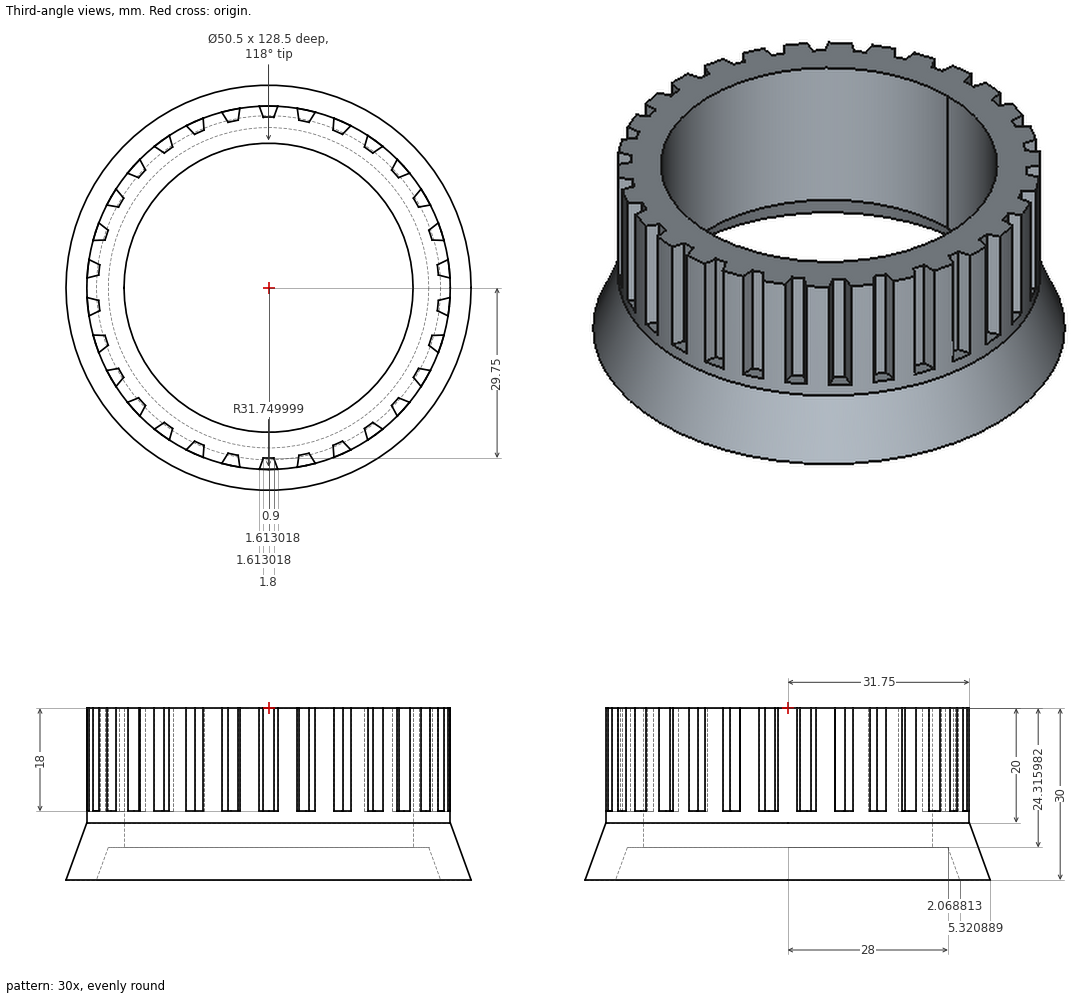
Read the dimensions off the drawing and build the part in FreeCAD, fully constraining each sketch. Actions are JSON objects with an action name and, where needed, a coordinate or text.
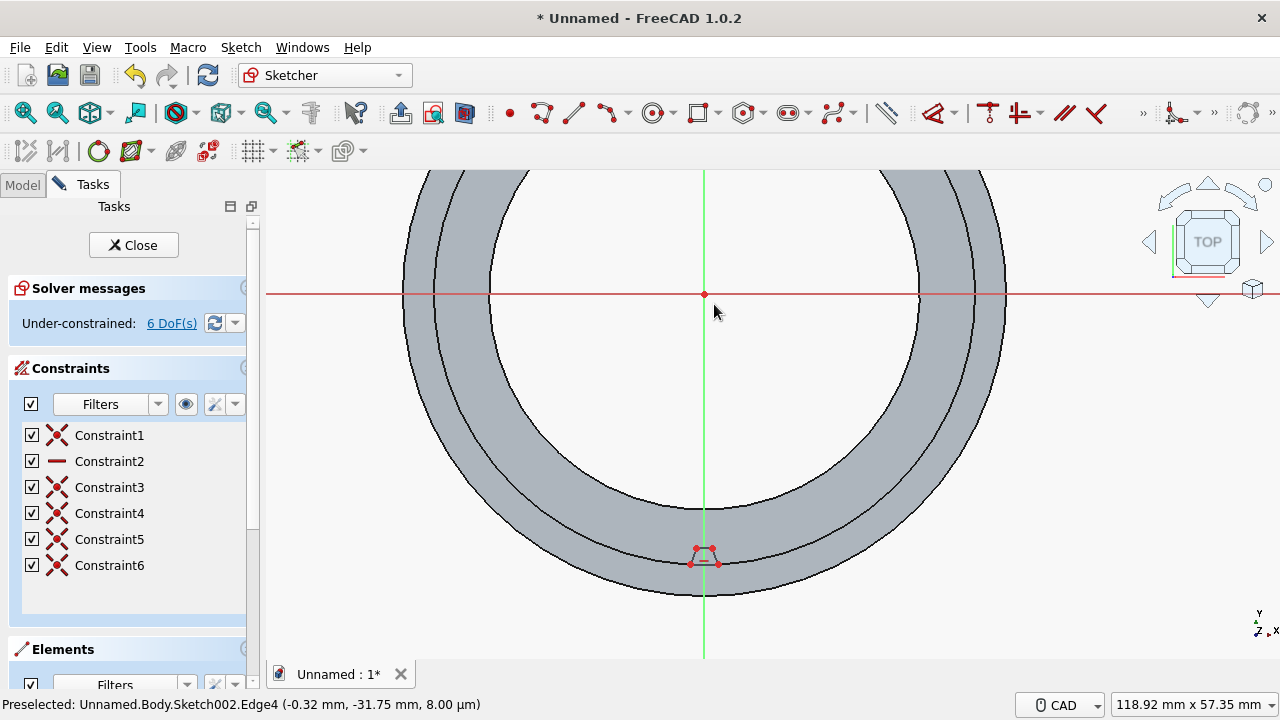
{"action": "left_click", "coordinate": [934, 114]}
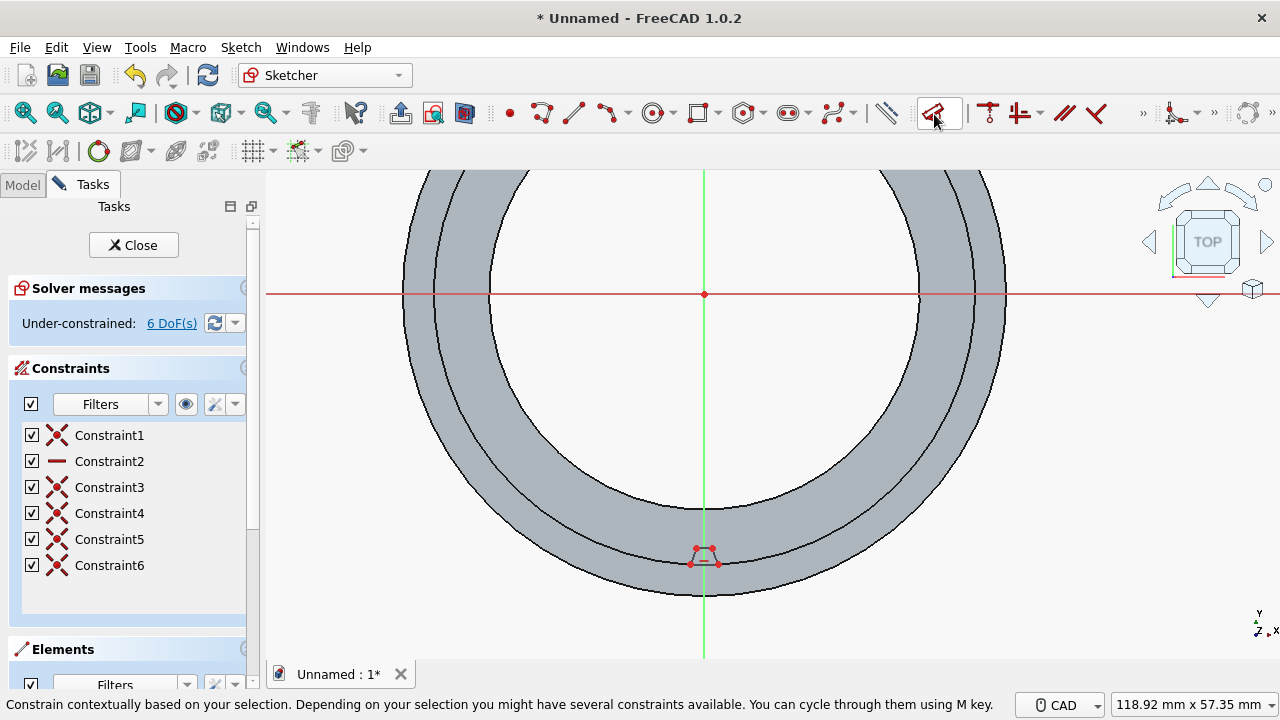
{"action": "left_click", "coordinate": [704, 565]}
{"action": "left_click", "coordinate": [559, 560]}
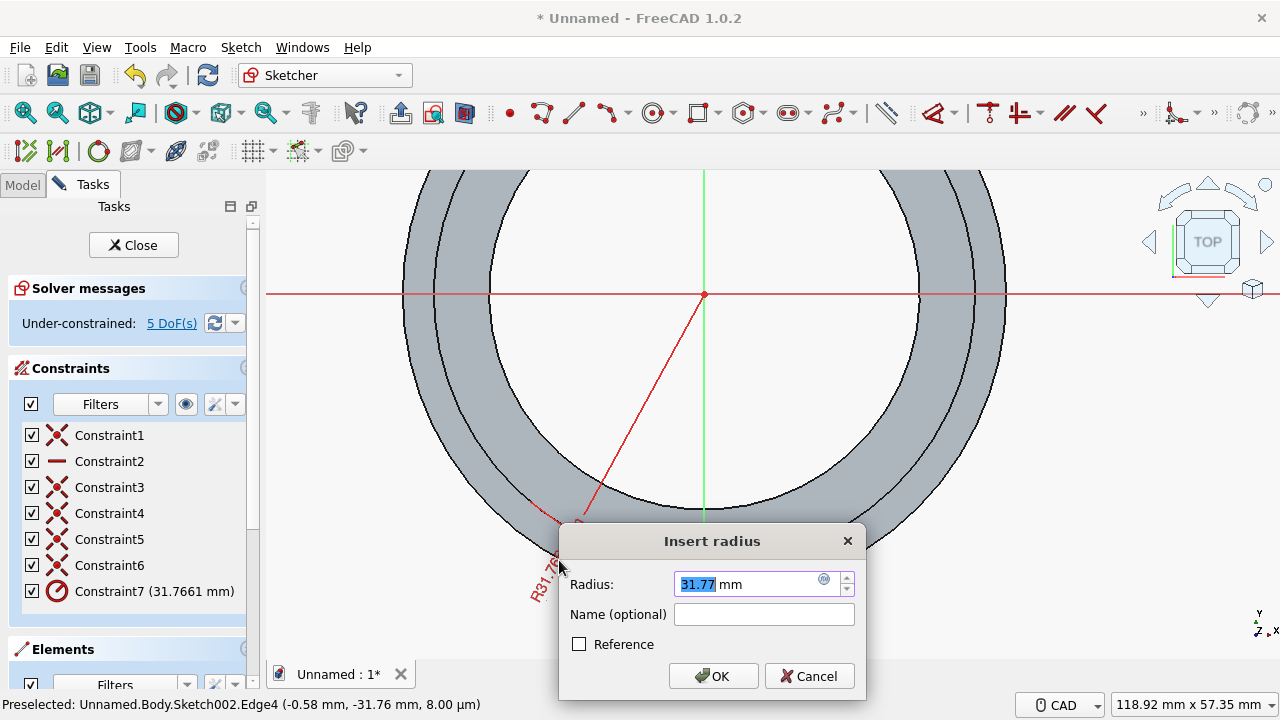
{"action": "type", "text": "31.749999"}
{"action": "key", "text": "Return"}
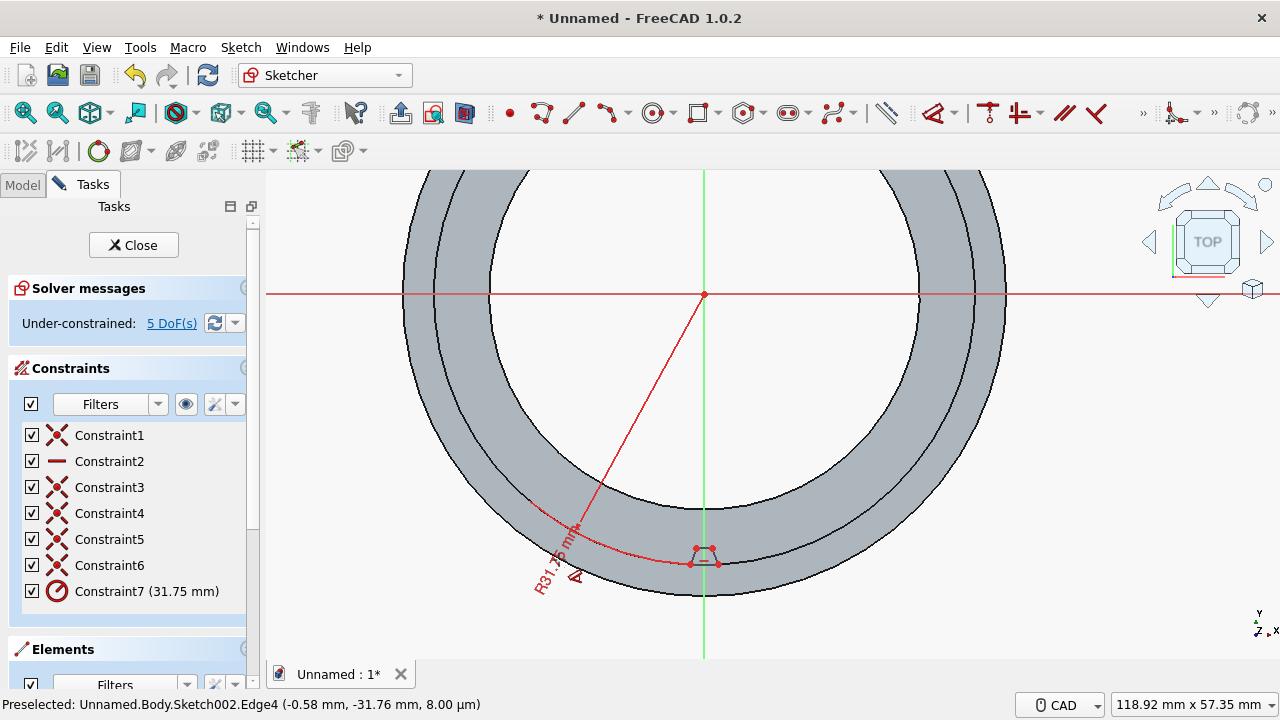
{"action": "scroll", "coordinate": [704, 548], "scroll_direction": "up", "scroll_amount": 5}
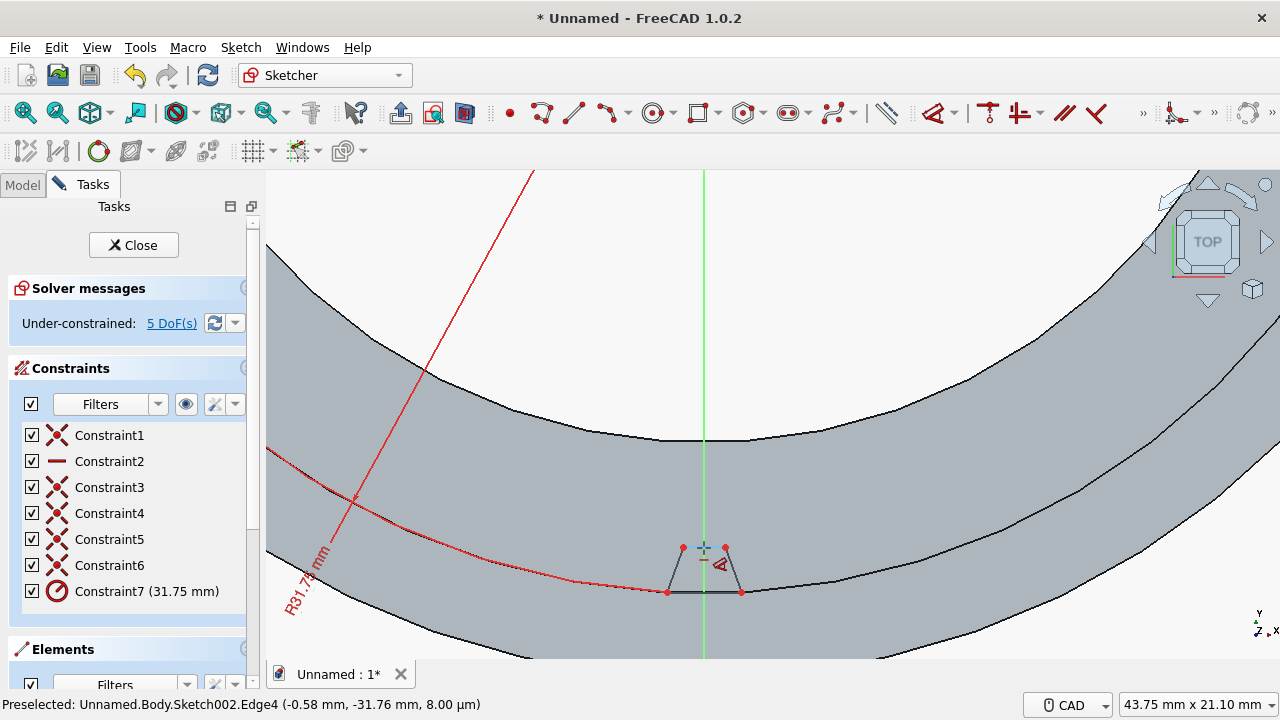
{"action": "left_click", "coordinate": [704, 547]}
{"action": "left_click", "coordinate": [690, 513]}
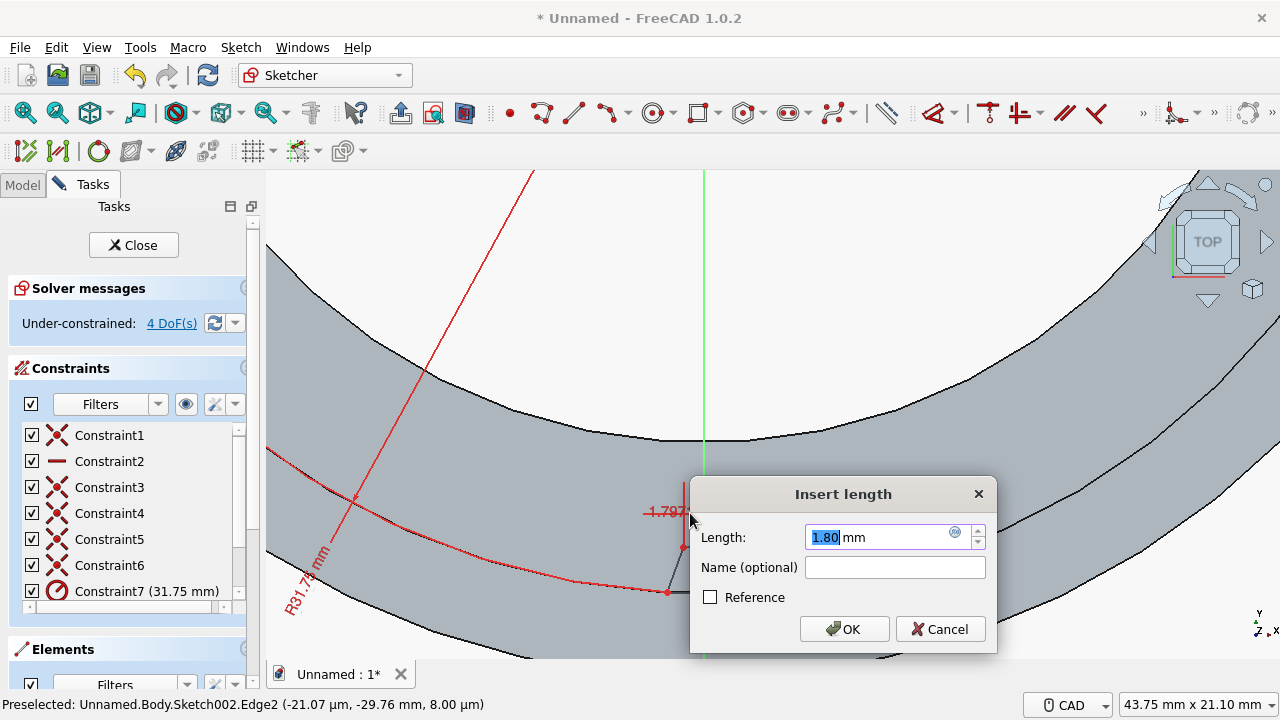
{"action": "type", "text": "1.8"}
{"action": "key", "text": "Return"}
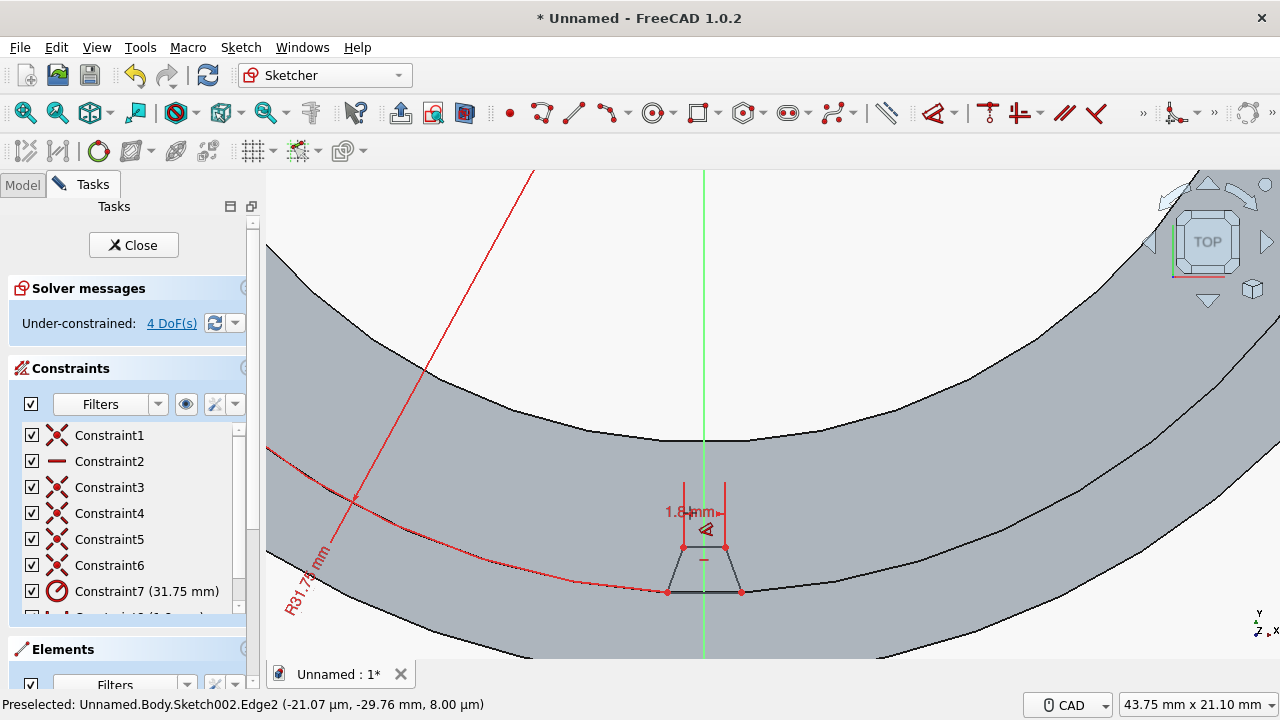
{"action": "scroll", "coordinate": [725, 547], "scroll_direction": "up", "scroll_amount": 4}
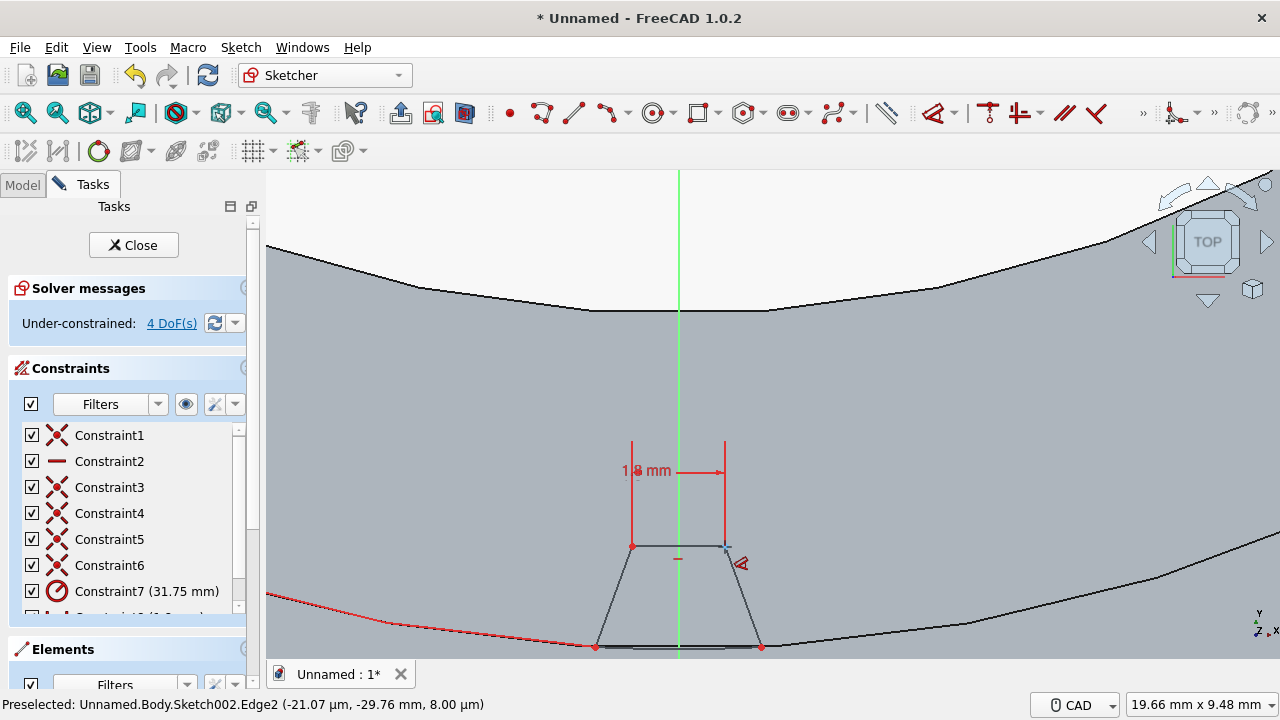
{"action": "left_click", "coordinate": [725, 546]}
{"action": "left_click", "coordinate": [702, 580]}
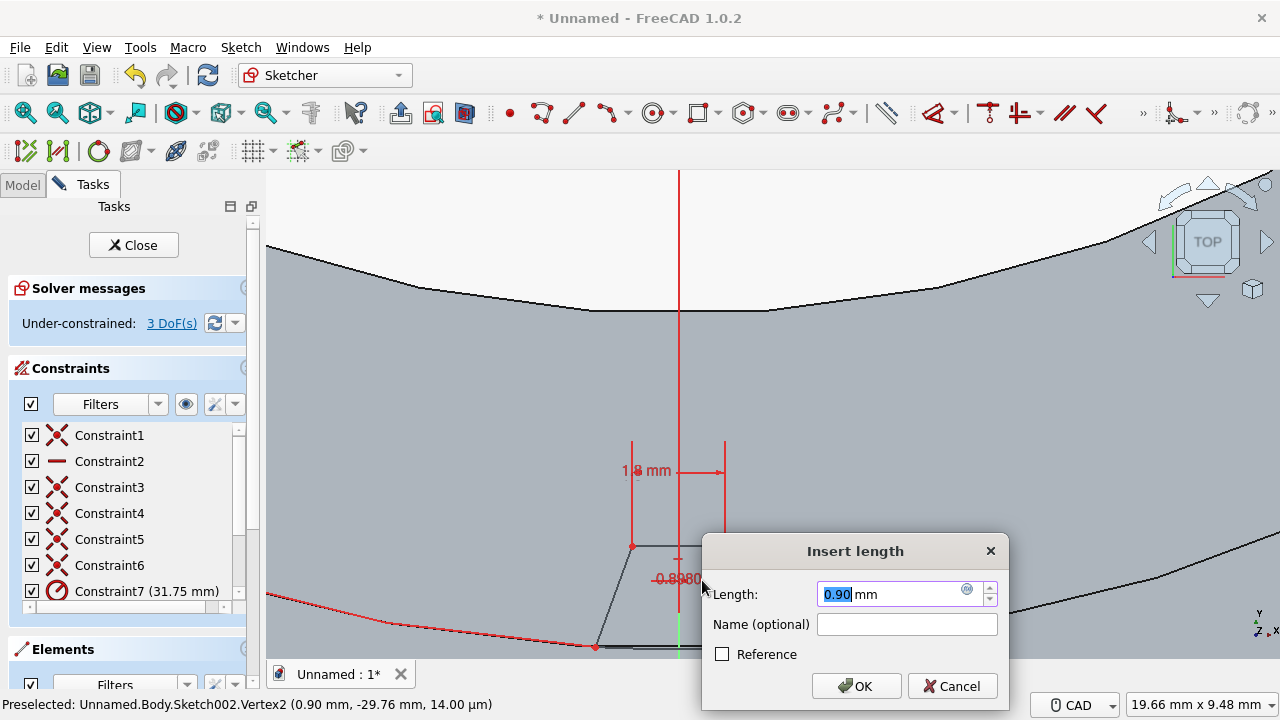
{"action": "type", "text": "0.9"}
{"action": "key", "text": "Return"}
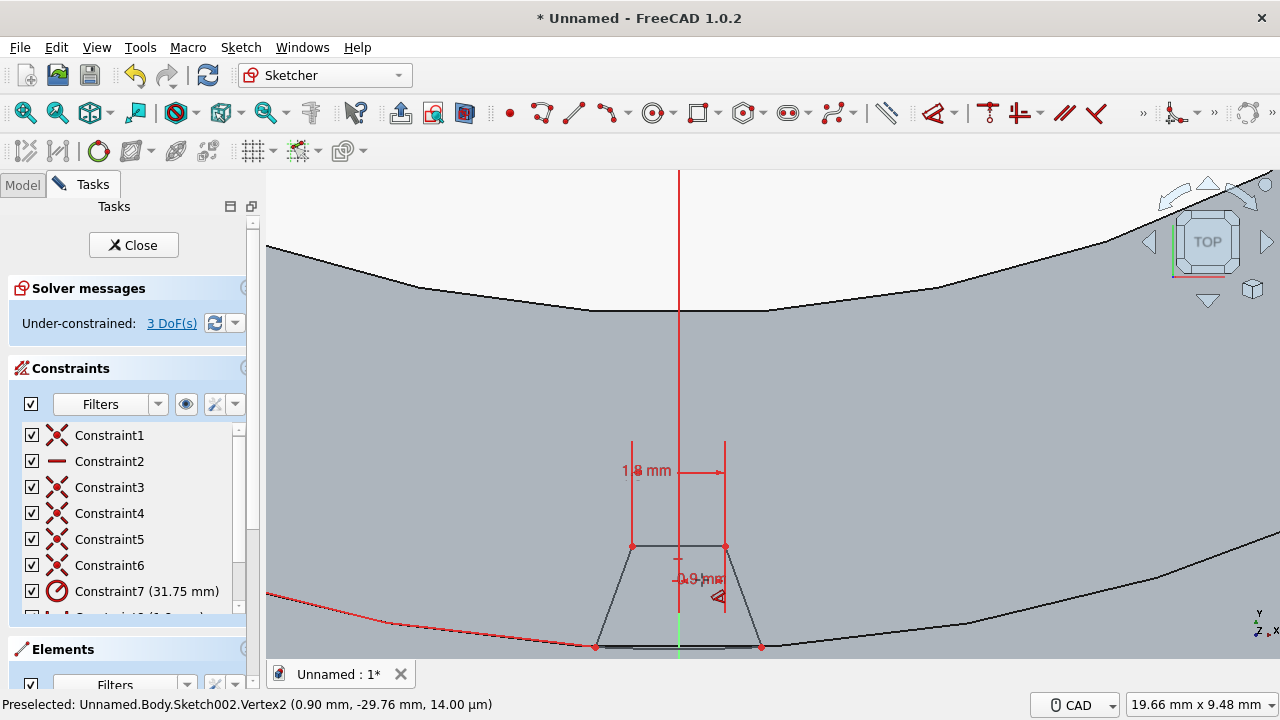
{"action": "left_click", "coordinate": [725, 546]}
{"action": "left_click", "coordinate": [759, 372]}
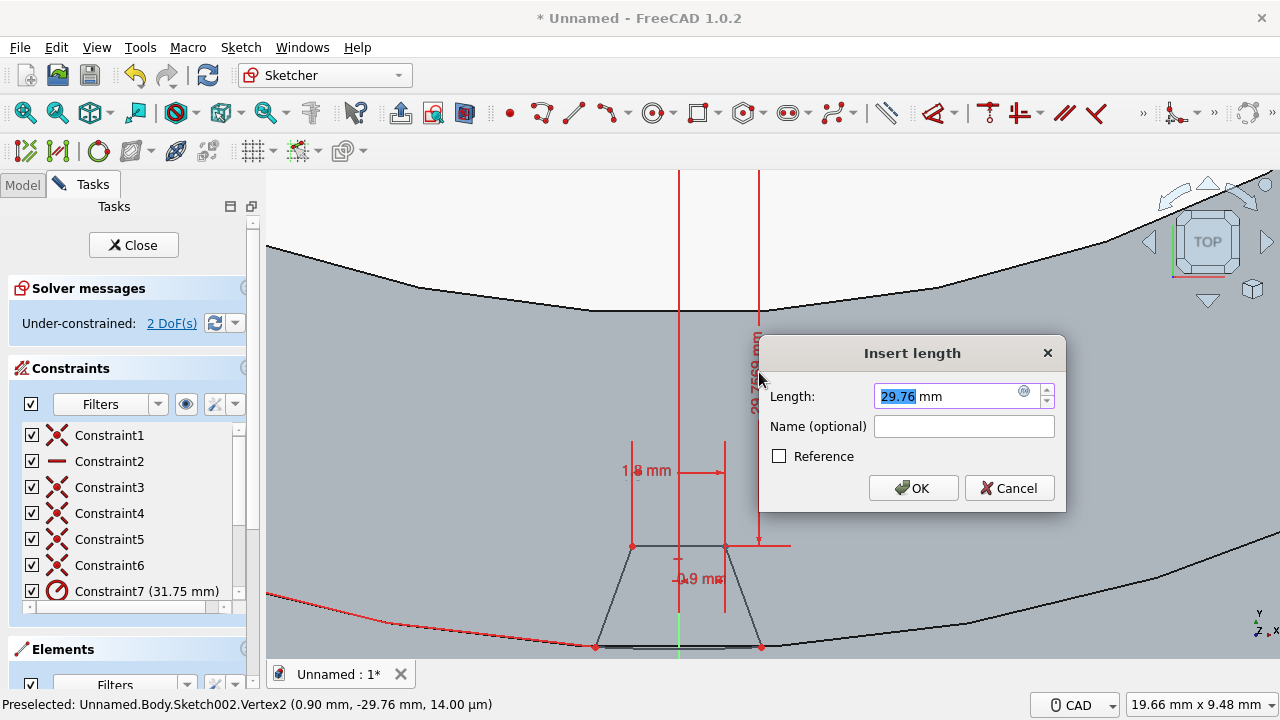
{"action": "type", "text": "29.75"}
{"action": "key", "text": "Return"}